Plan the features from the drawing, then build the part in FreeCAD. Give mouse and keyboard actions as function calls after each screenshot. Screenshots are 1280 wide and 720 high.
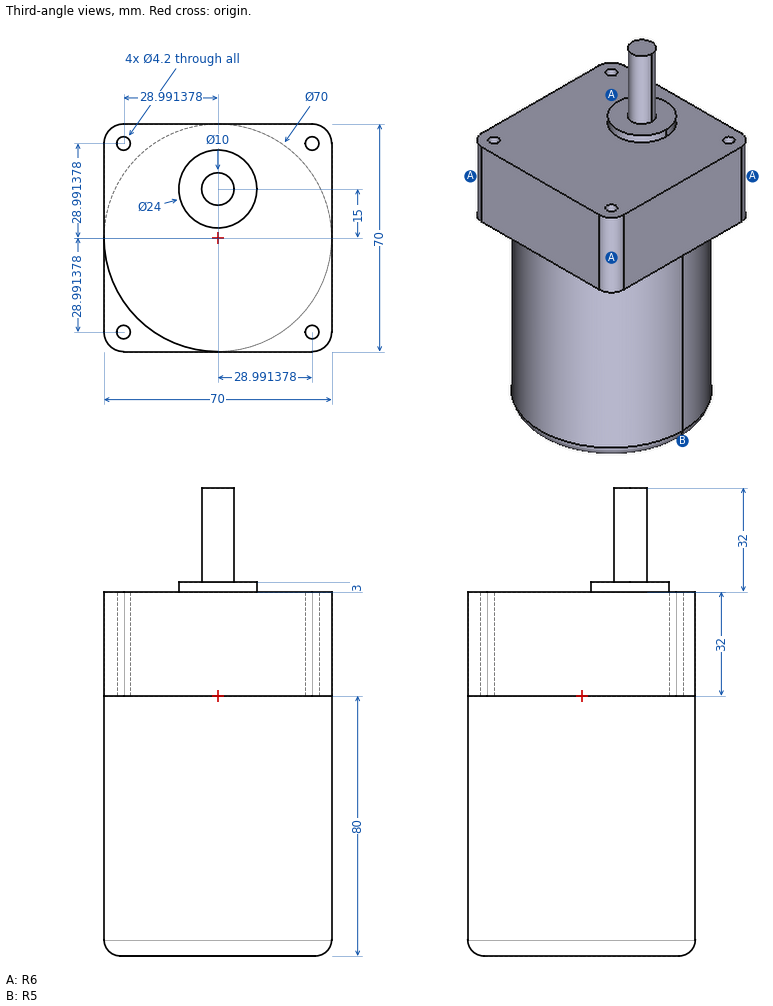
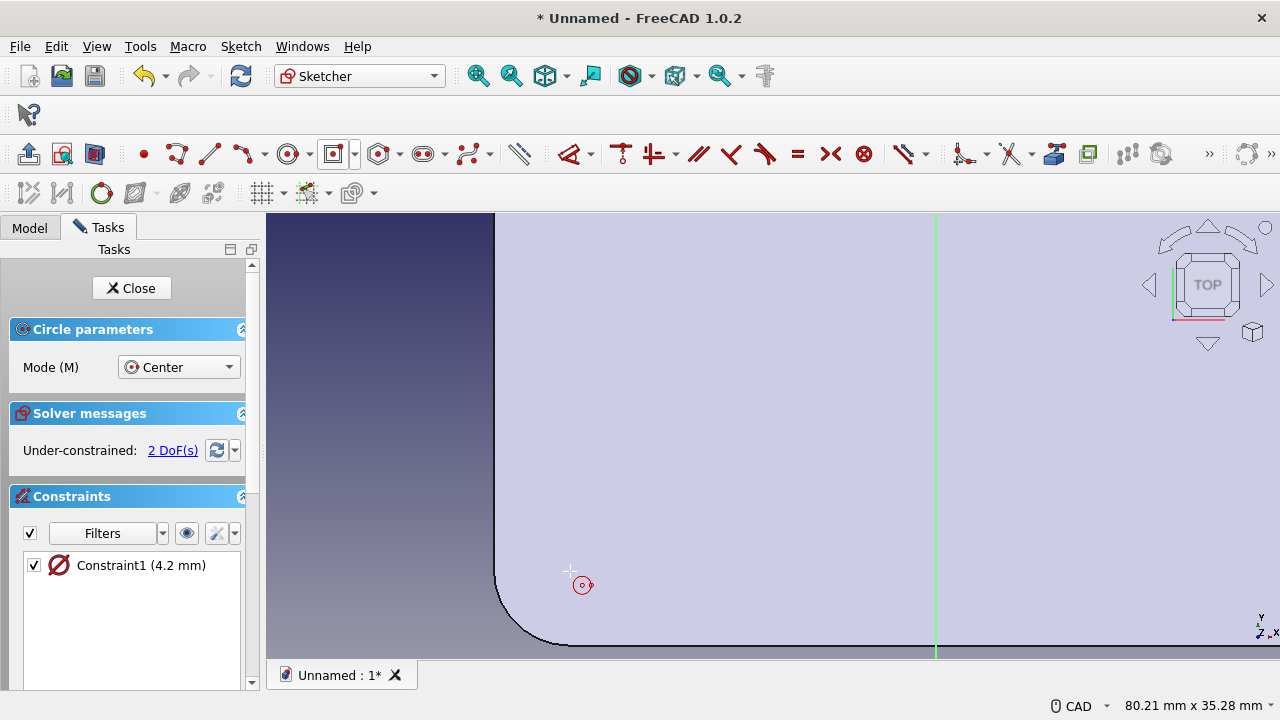
click(570, 570)
move(589, 551)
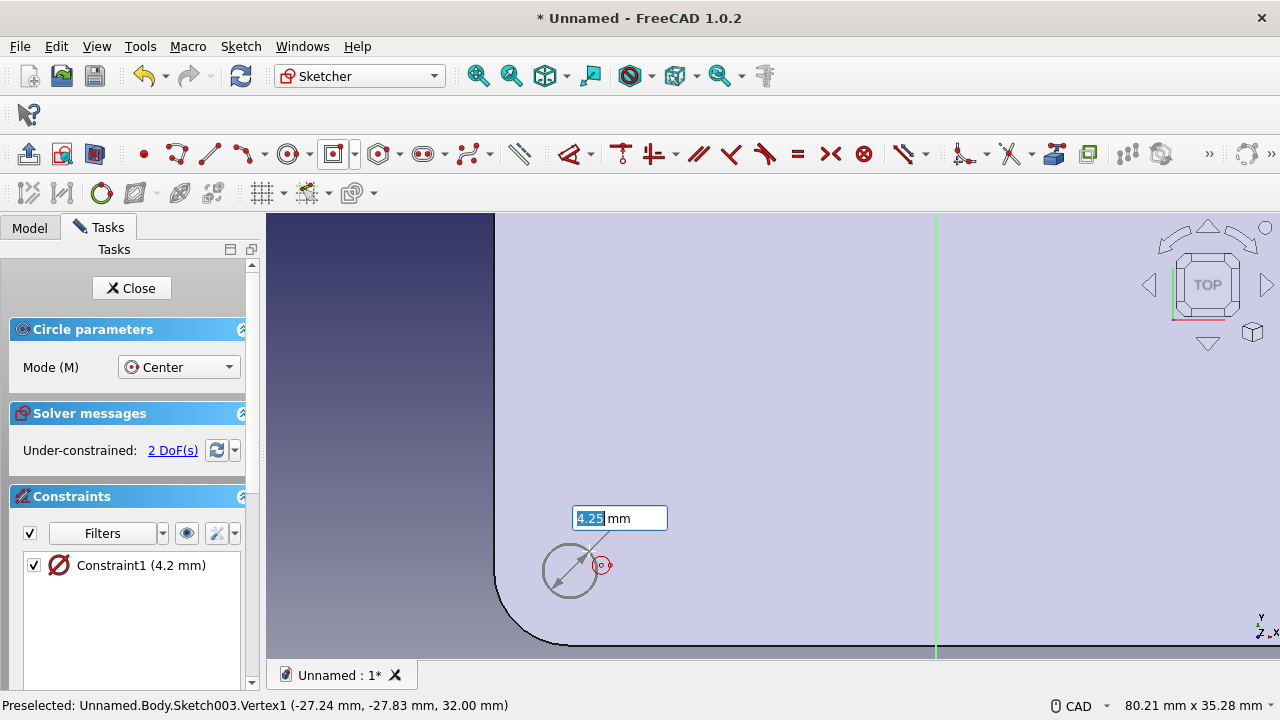
text(4.2)
key(Return)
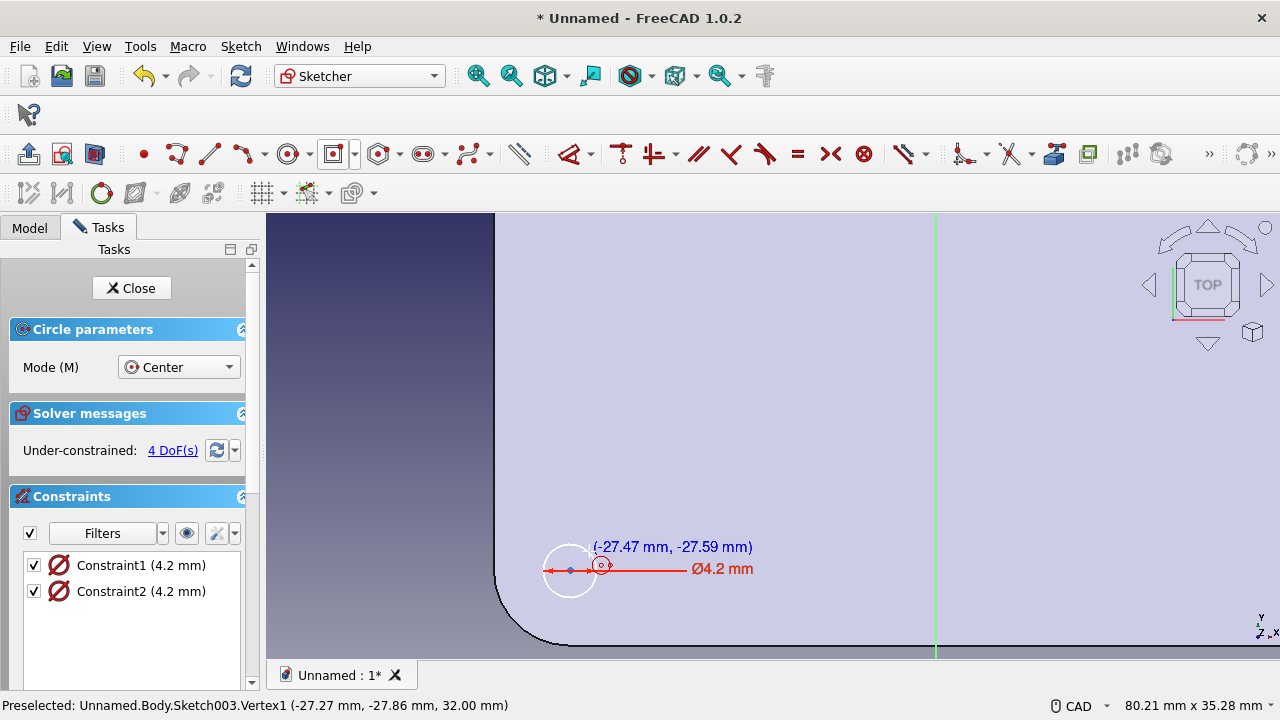
scroll(570, 571, down, 5)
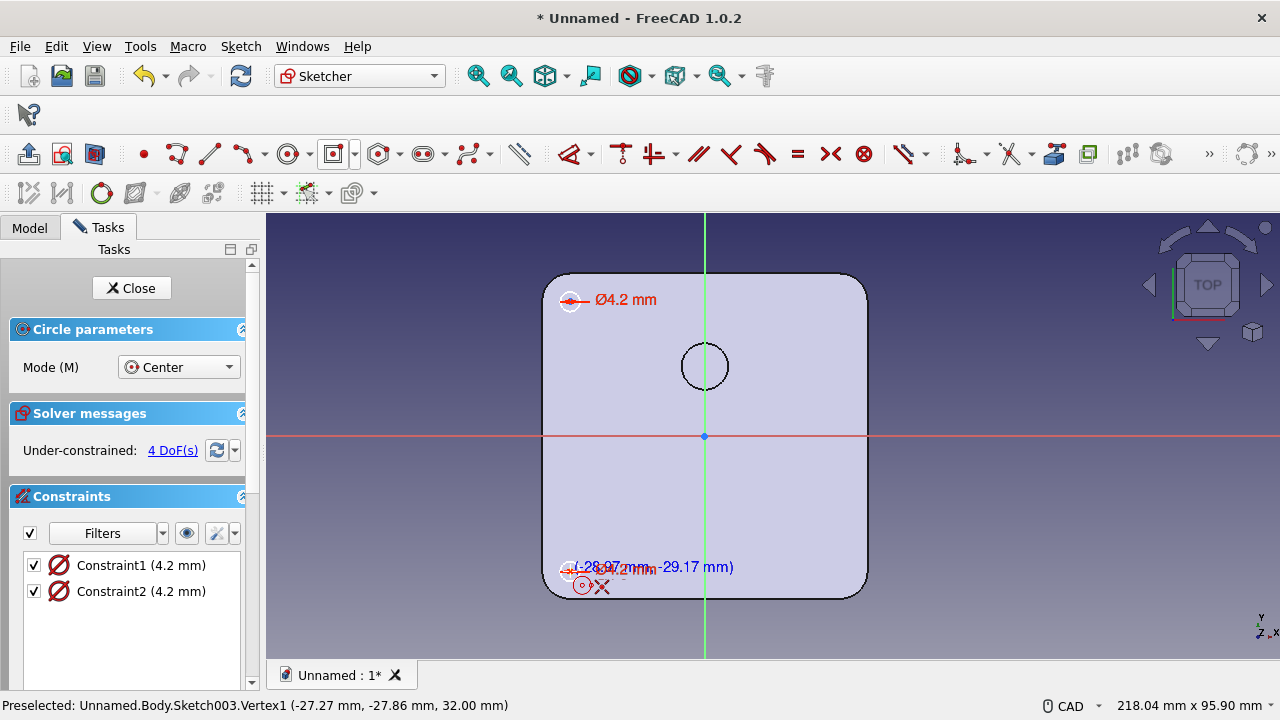
scroll(840, 571, up, 5)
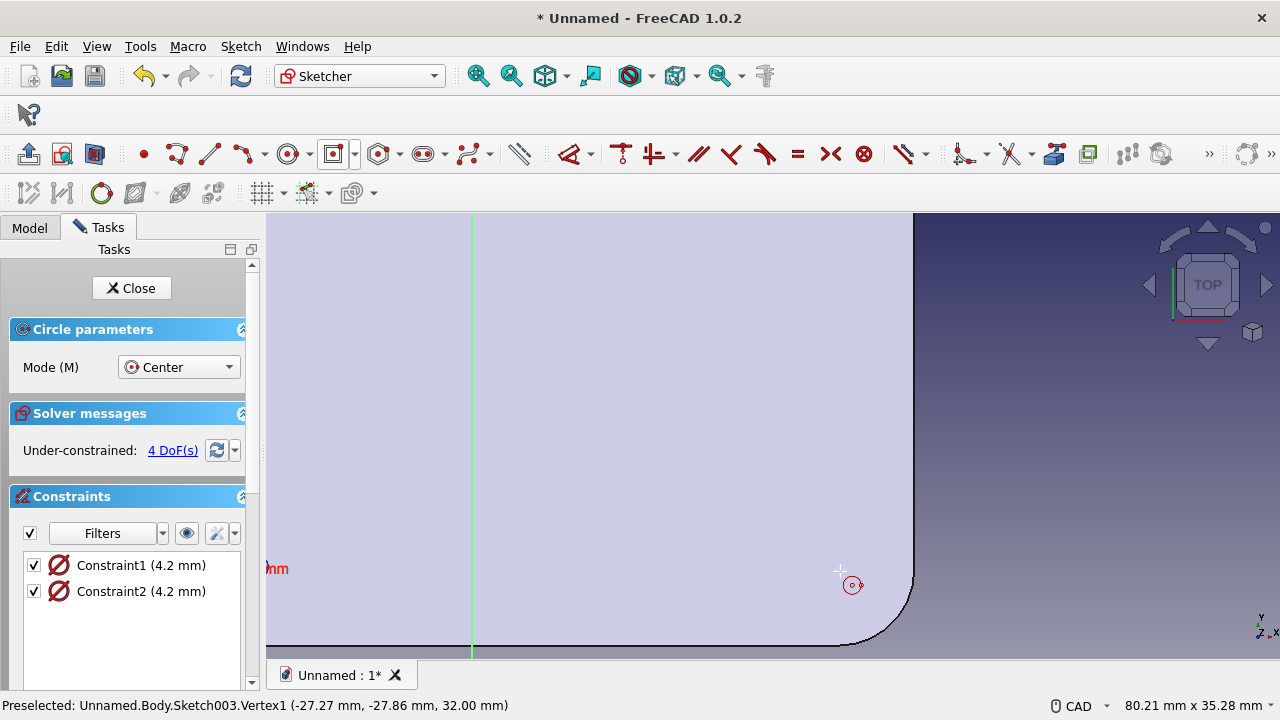
click(838, 570)
move(857, 551)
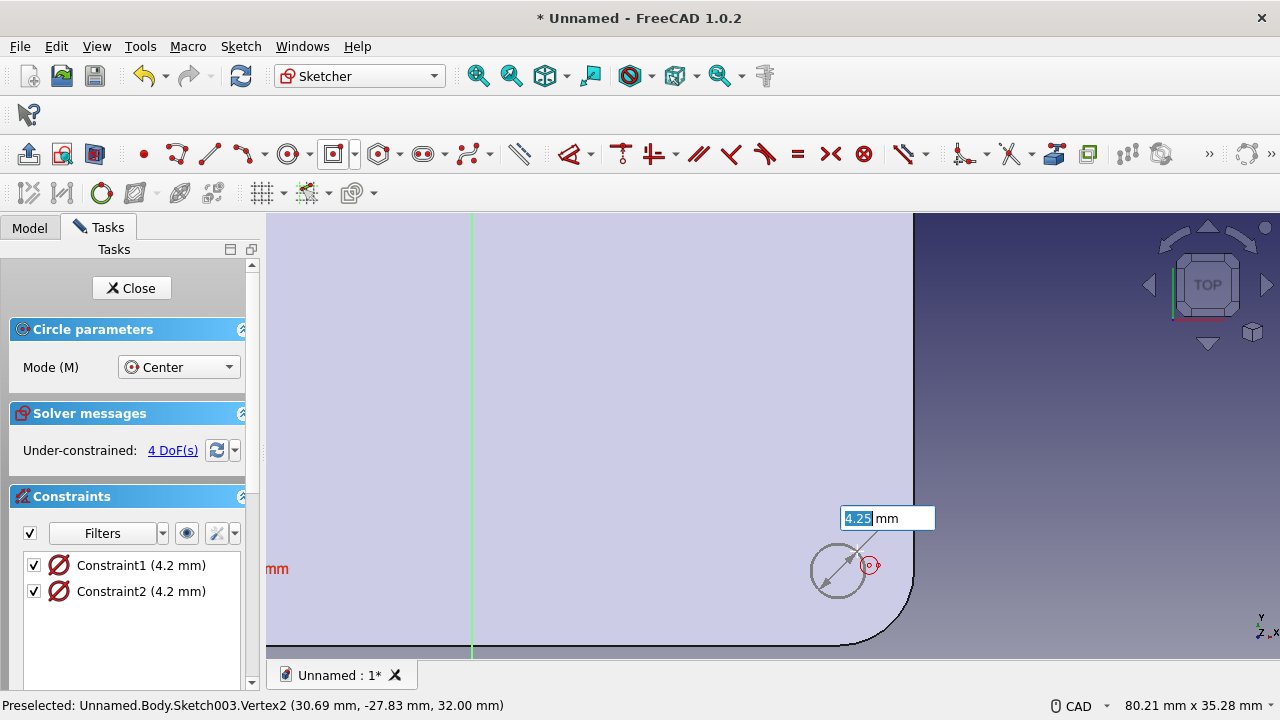
text(4.2)
key(Return)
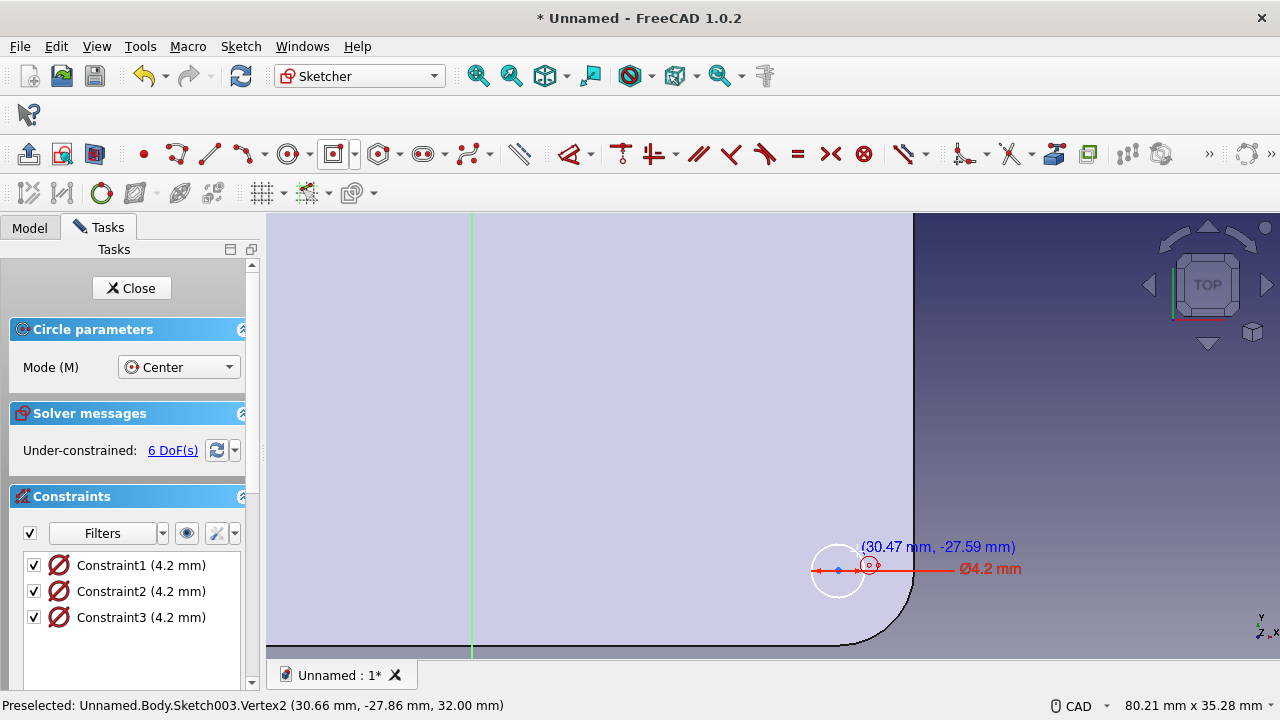
scroll(840, 571, down, 5)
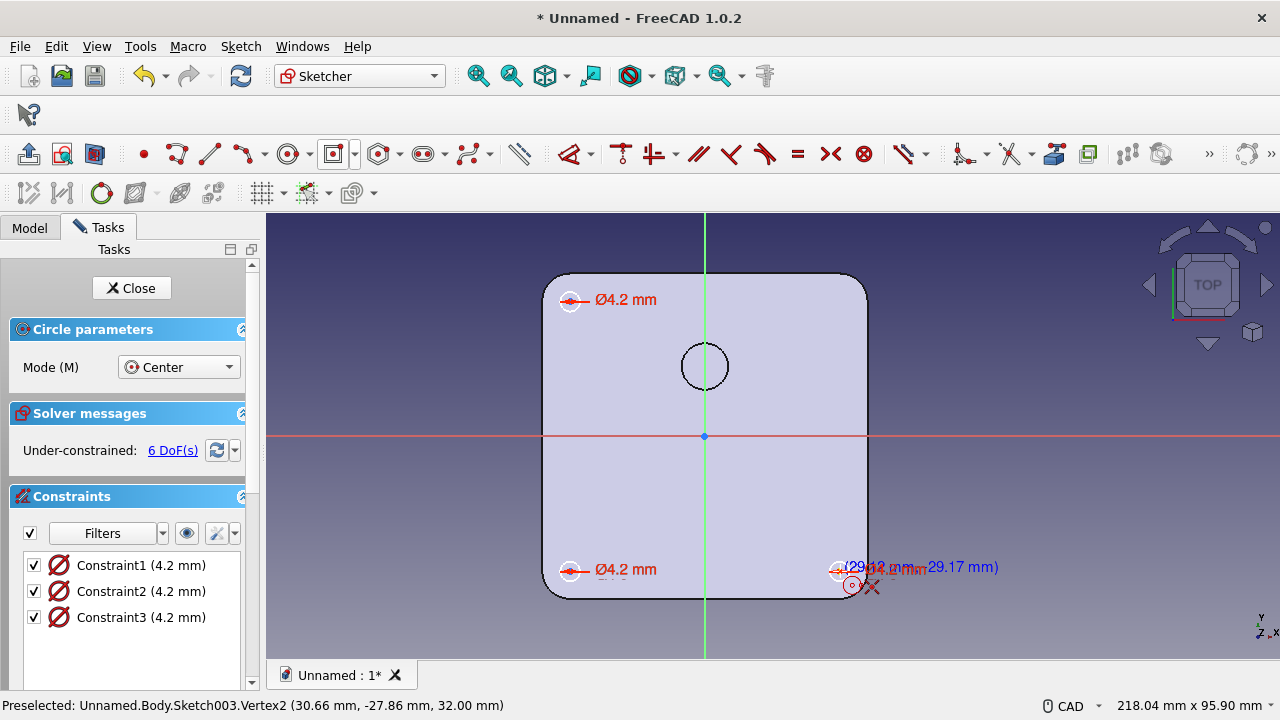
scroll(840, 301, up, 5)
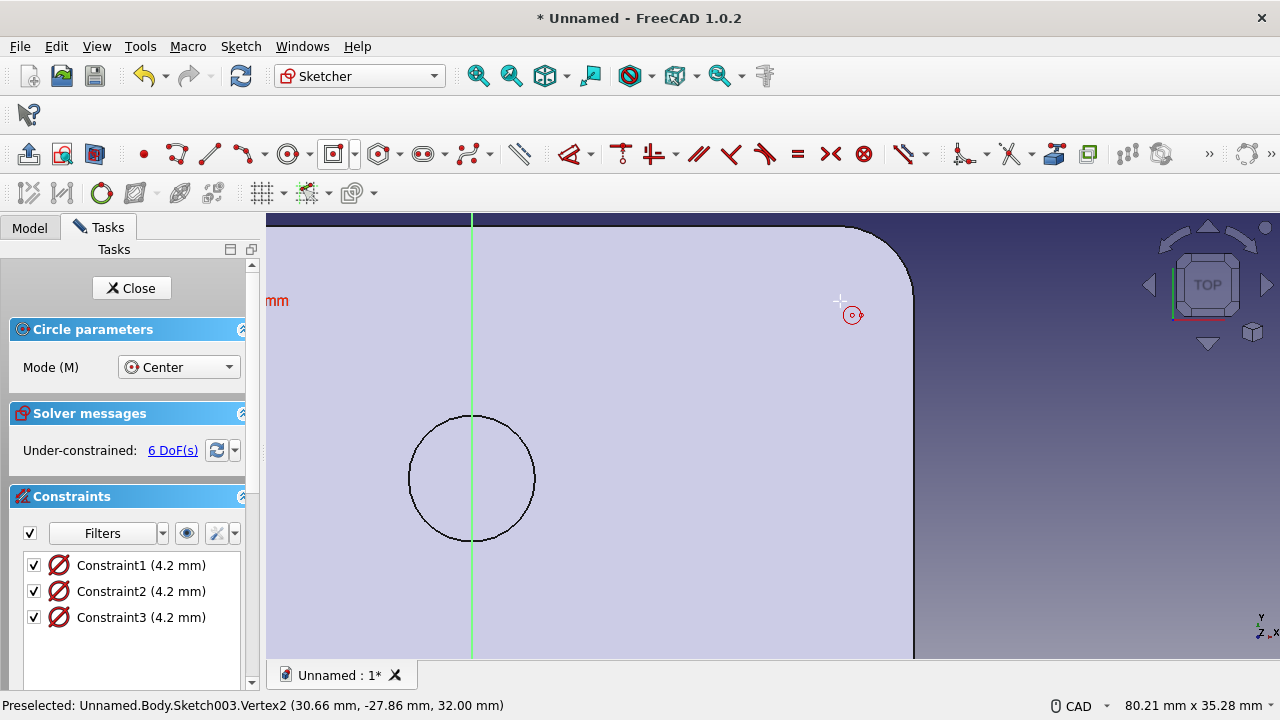
click(838, 302)
move(857, 283)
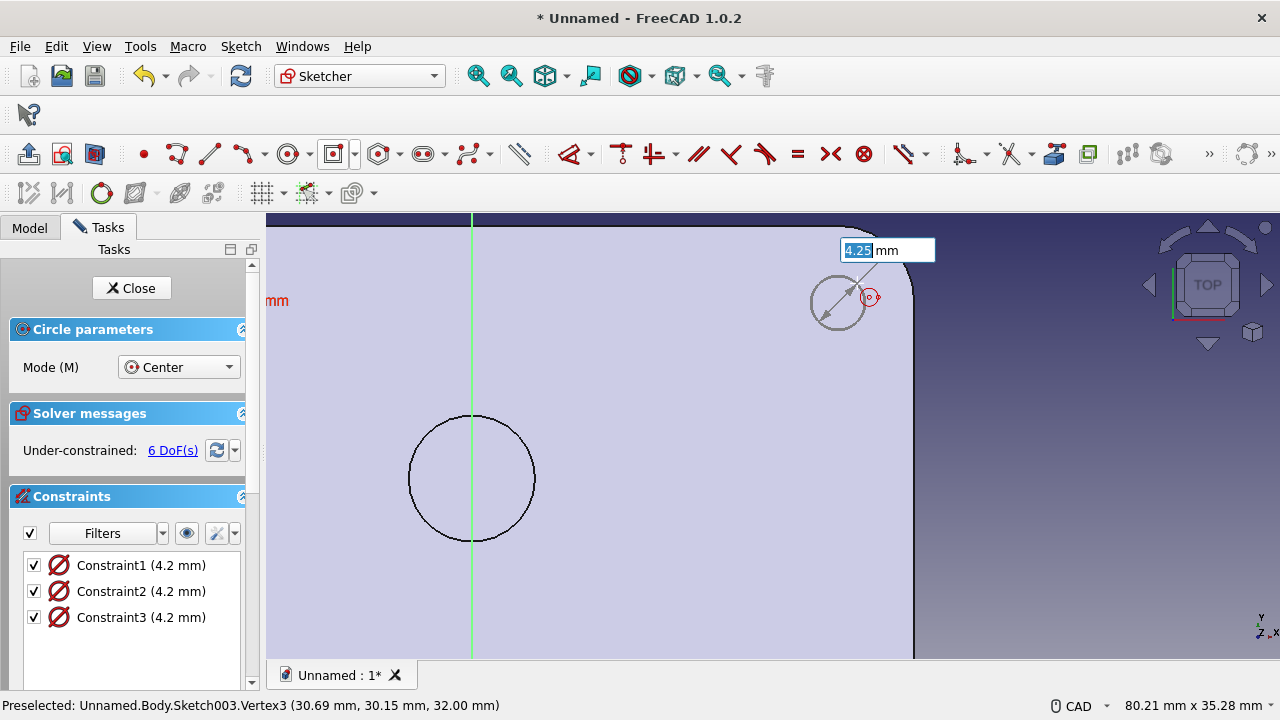
text(4.2)
key(Return)
key(Escape)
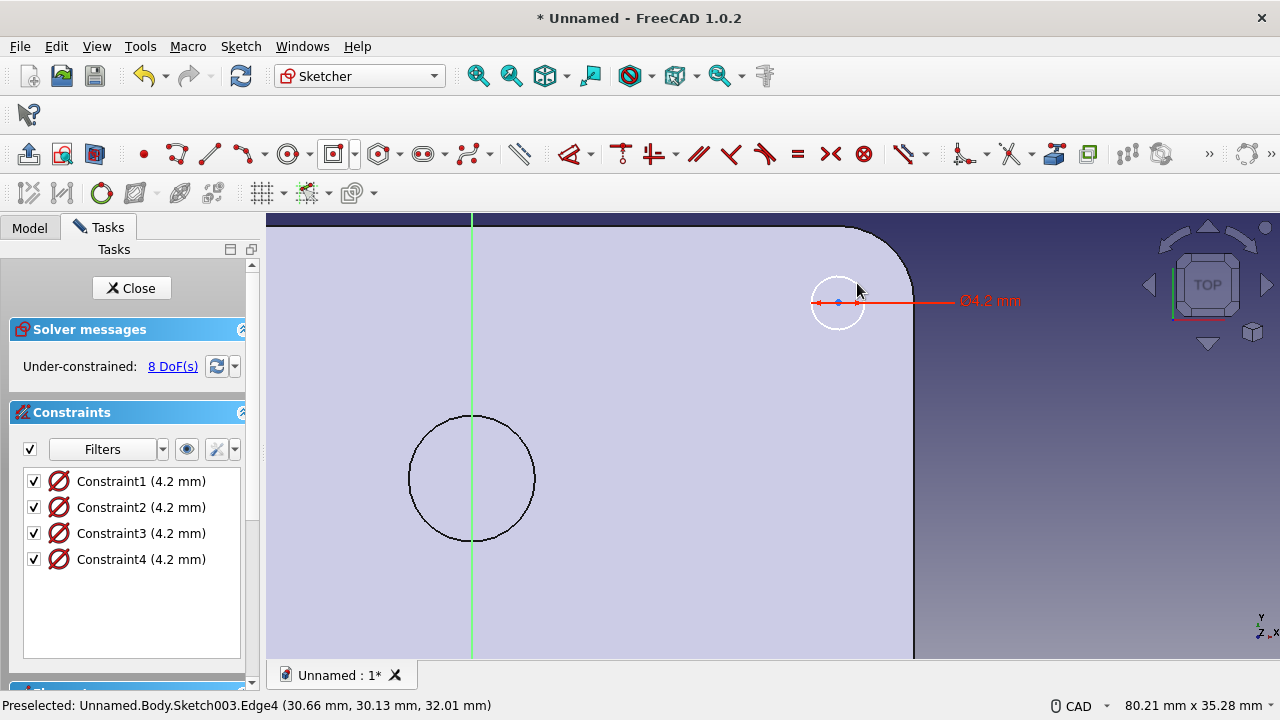
scroll(840, 301, down, 5)